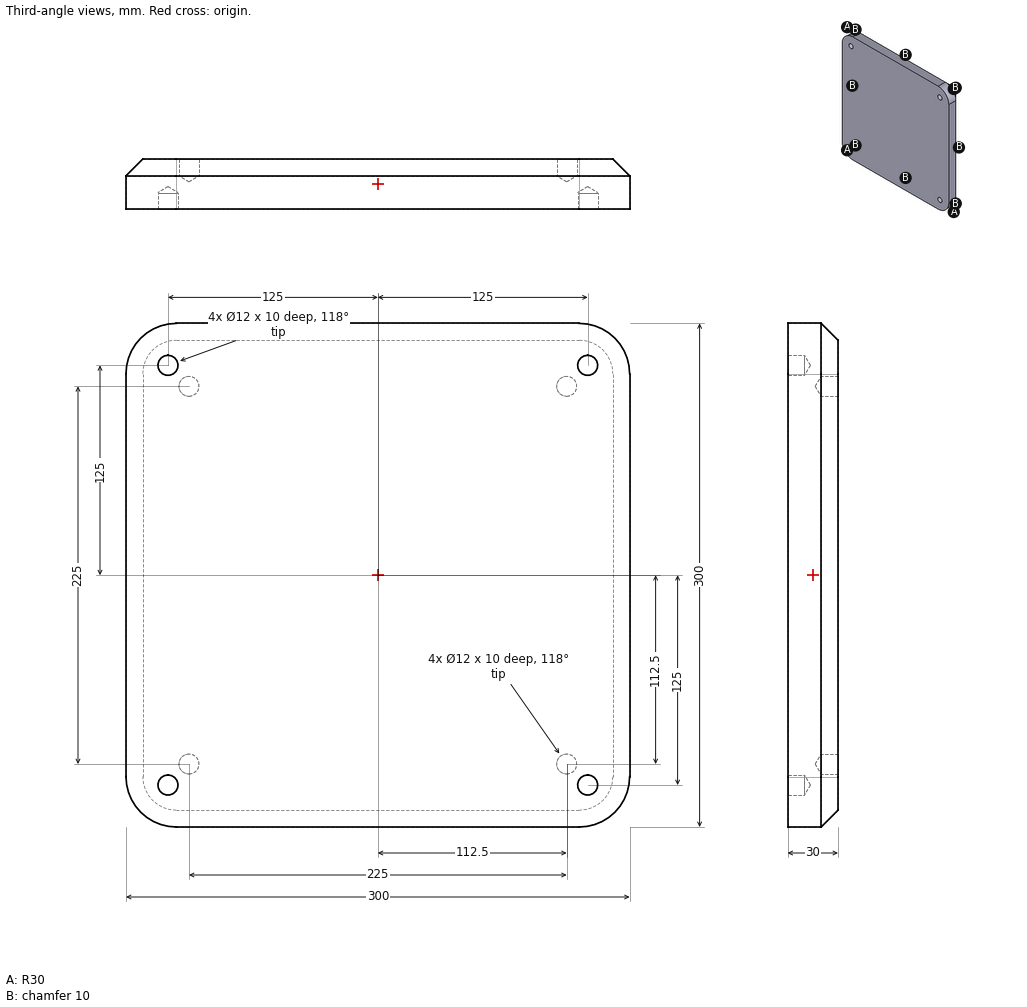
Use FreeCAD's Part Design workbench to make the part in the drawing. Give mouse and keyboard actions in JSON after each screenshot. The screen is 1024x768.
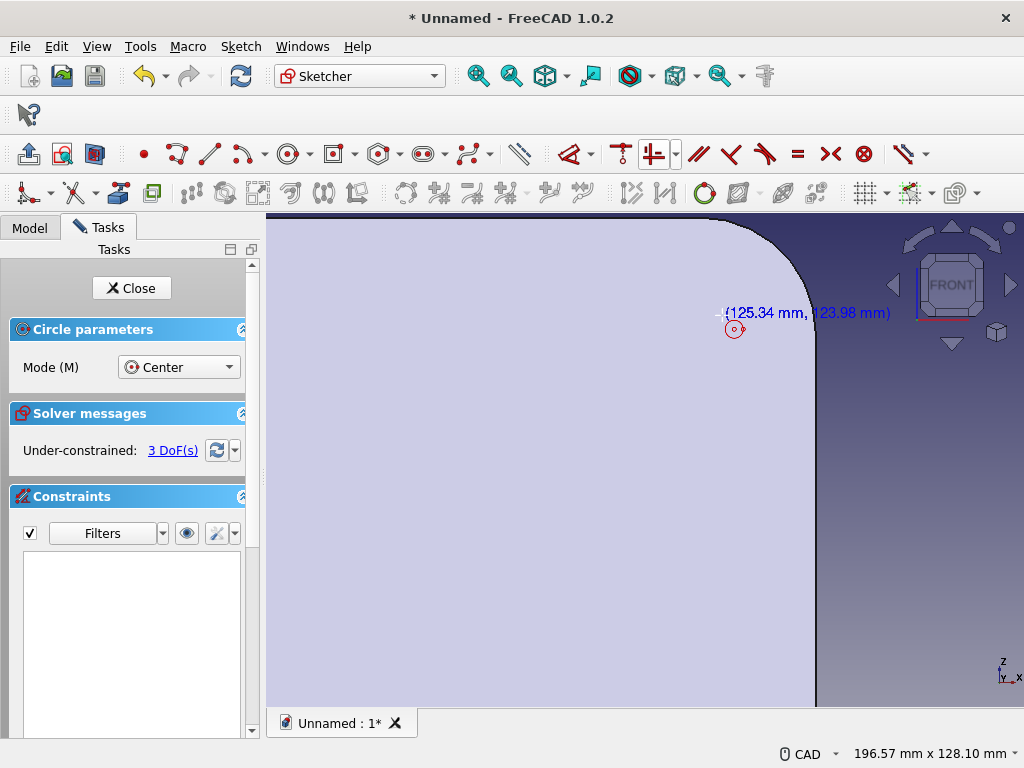
{"action": "left_click", "coordinate": [719, 314]}
{"action": "left_click", "coordinate": [736, 298]}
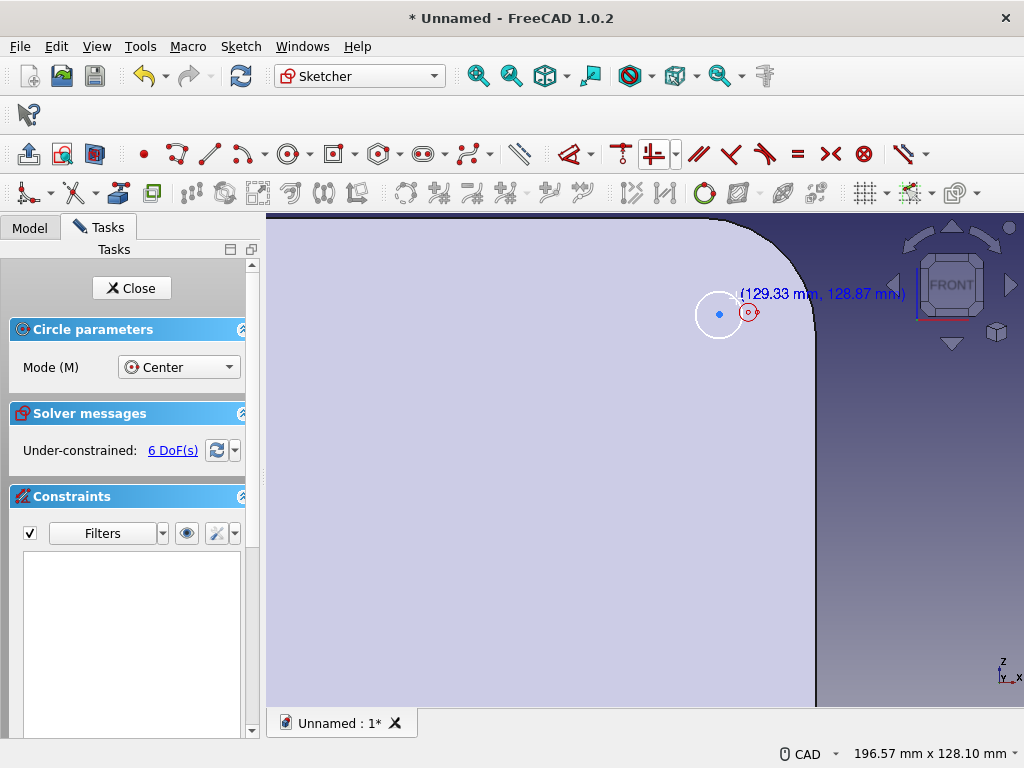
{"action": "scroll", "coordinate": [723, 315], "scroll_direction": "down", "scroll_amount": 6}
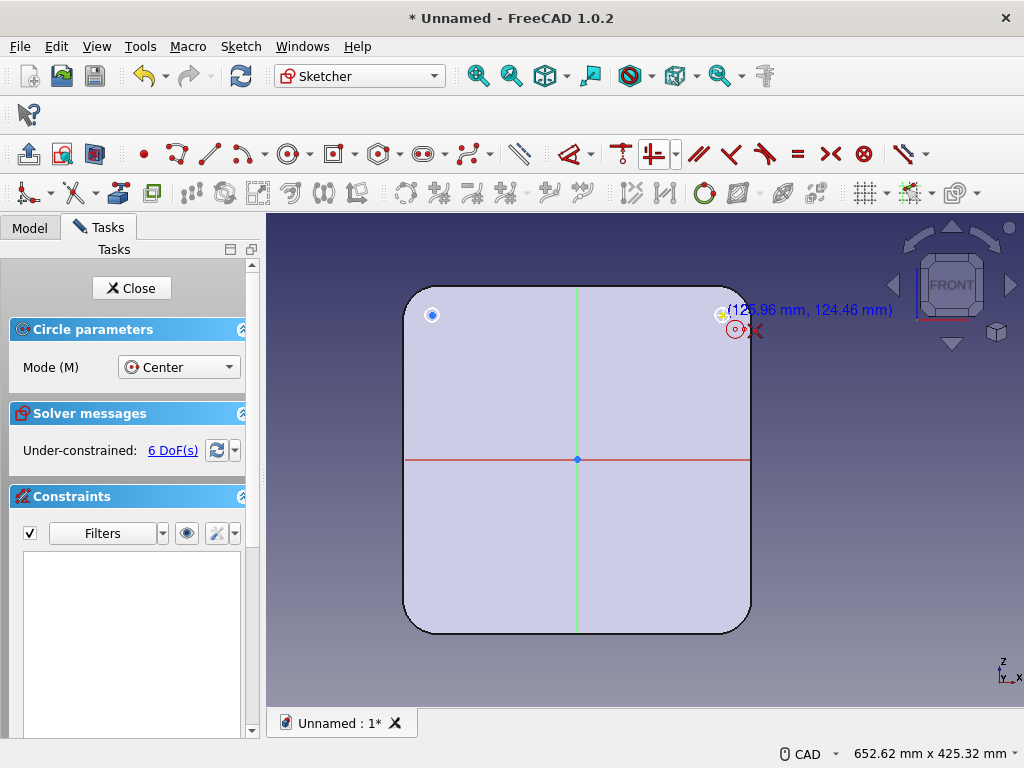
{"action": "scroll", "coordinate": [722, 605], "scroll_direction": "up", "scroll_amount": 6}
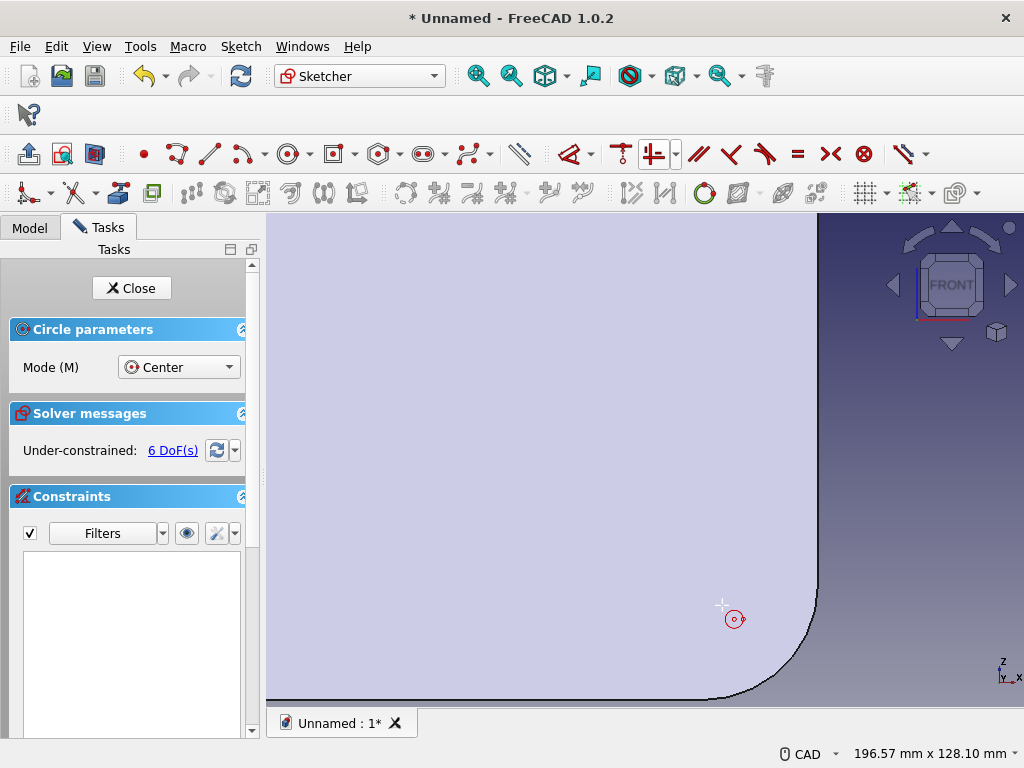
{"action": "left_click", "coordinate": [722, 604]}
{"action": "left_click", "coordinate": [738, 587]}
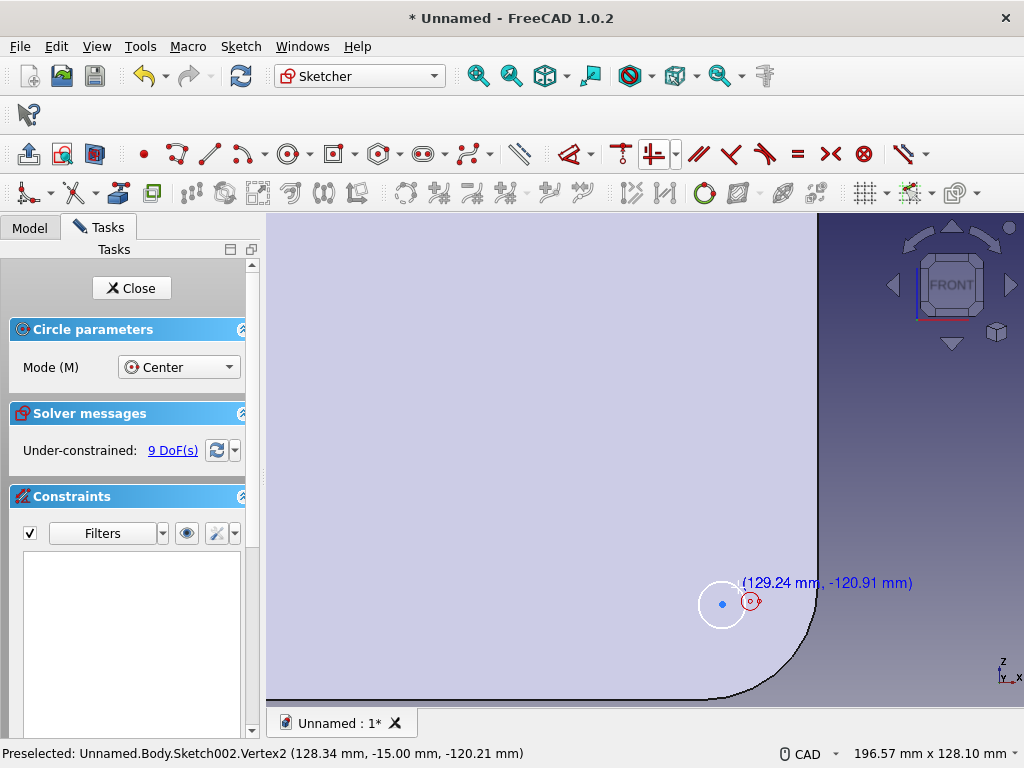
{"action": "scroll", "coordinate": [722, 606], "scroll_direction": "down", "scroll_amount": 6}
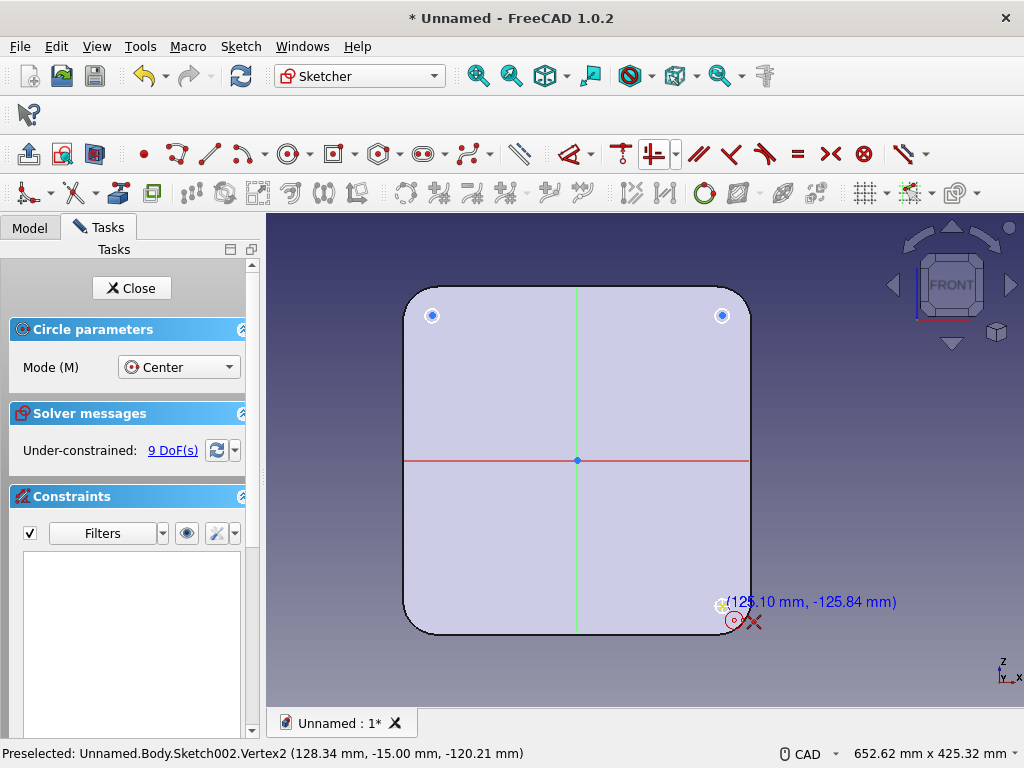
{"action": "scroll", "coordinate": [432, 606], "scroll_direction": "up", "scroll_amount": 6}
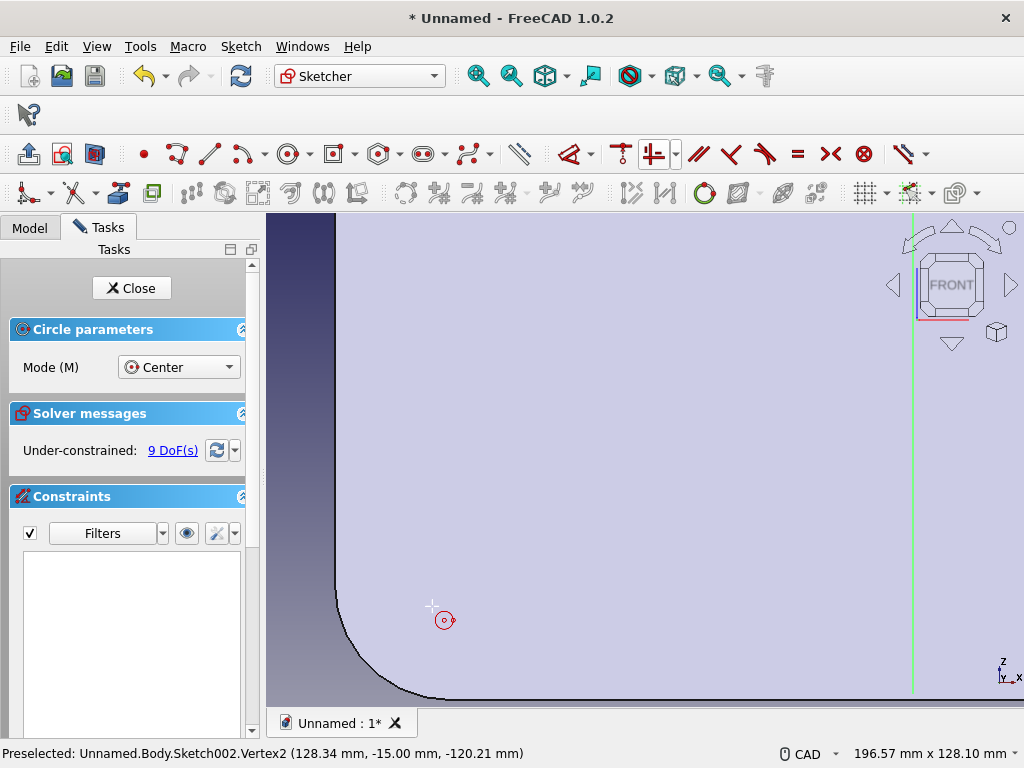
{"action": "left_click", "coordinate": [431, 604]}
{"action": "left_click", "coordinate": [448, 587]}
{"action": "key", "text": "Escape"}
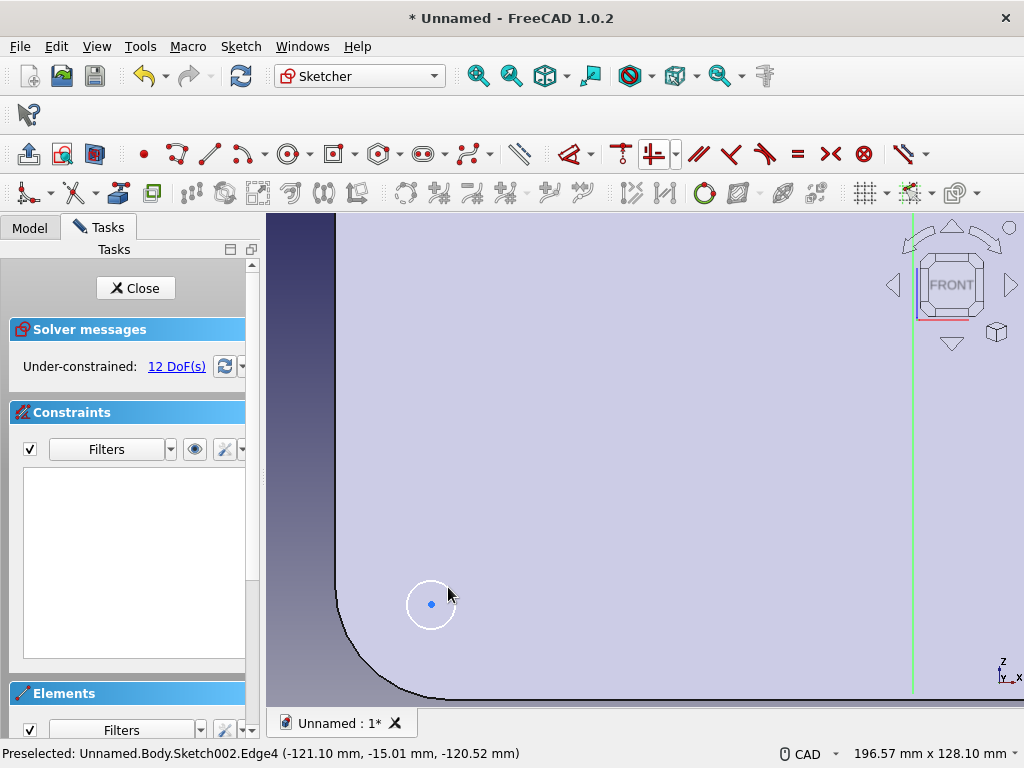
{"action": "scroll", "coordinate": [431, 606], "scroll_direction": "down", "scroll_amount": 6}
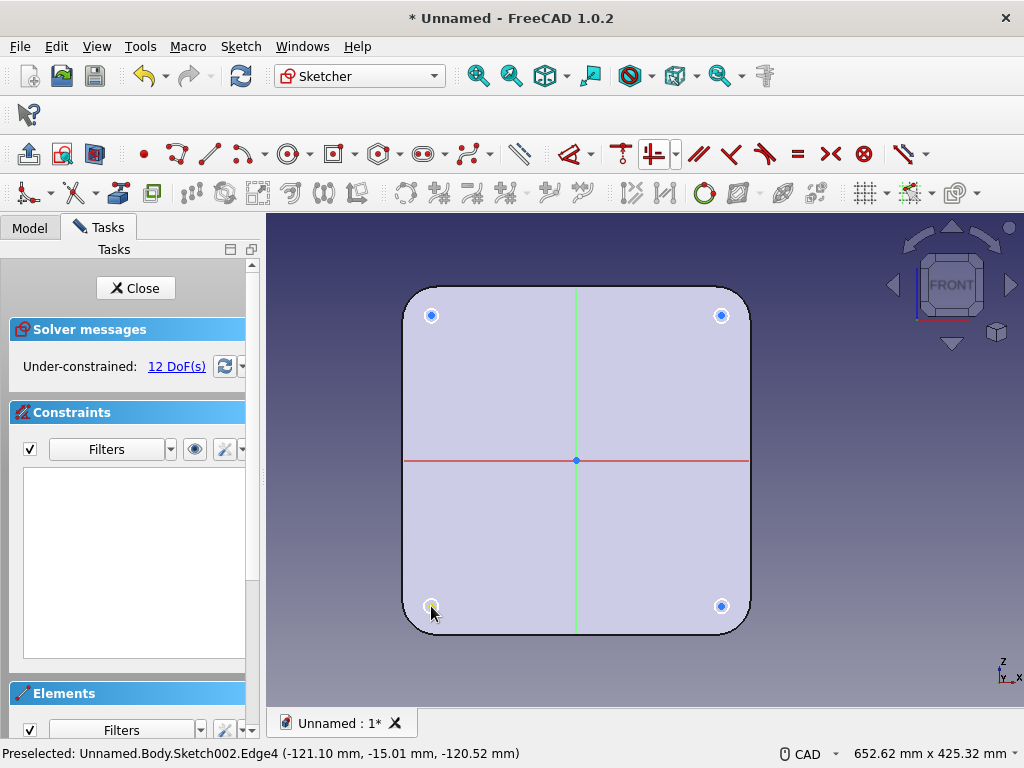
{"action": "scroll", "coordinate": [436, 311], "scroll_direction": "up", "scroll_amount": 4}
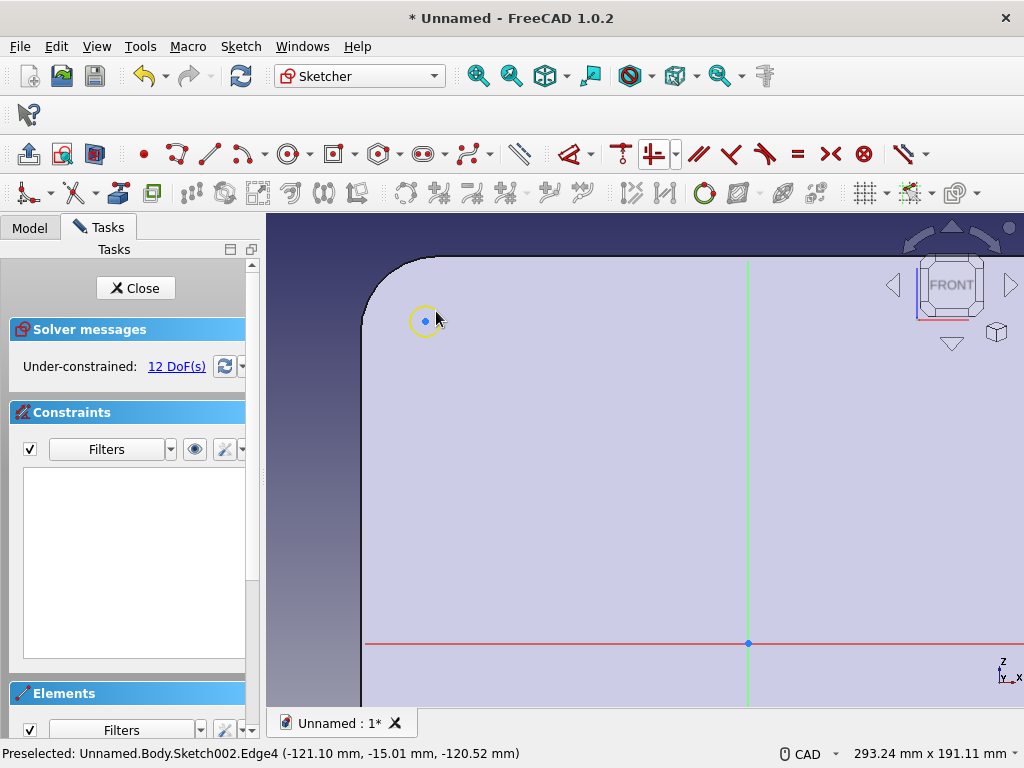
{"action": "left_click", "coordinate": [436, 311]}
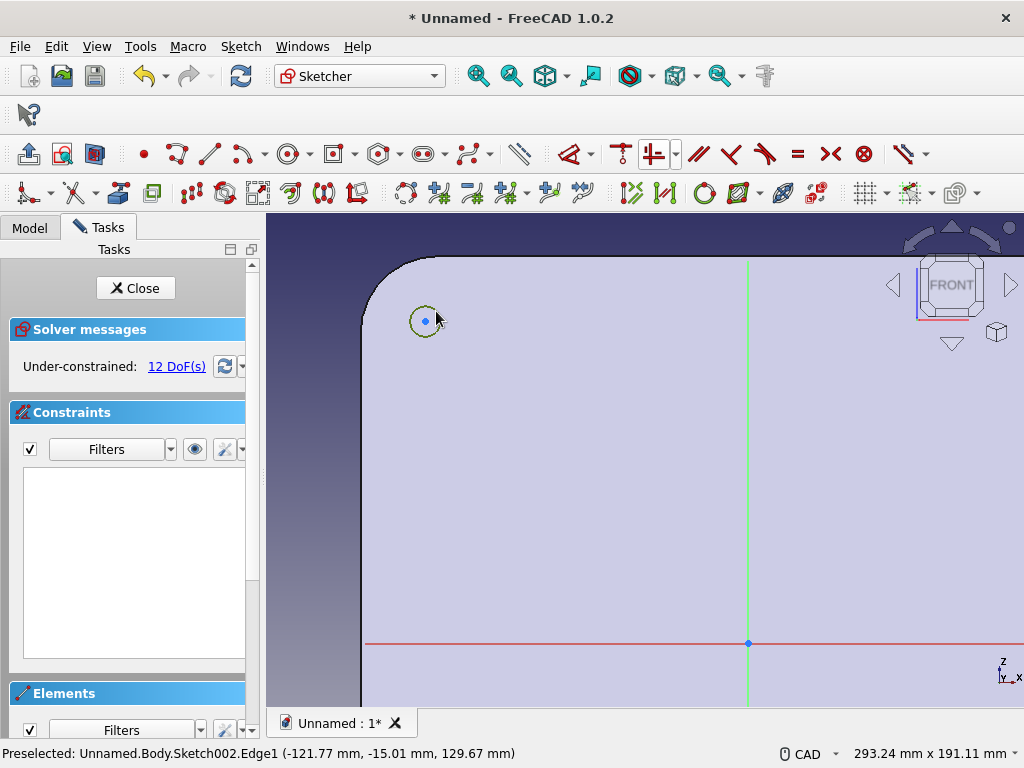
{"action": "scroll", "coordinate": [436, 310], "scroll_direction": "down", "scroll_amount": 4}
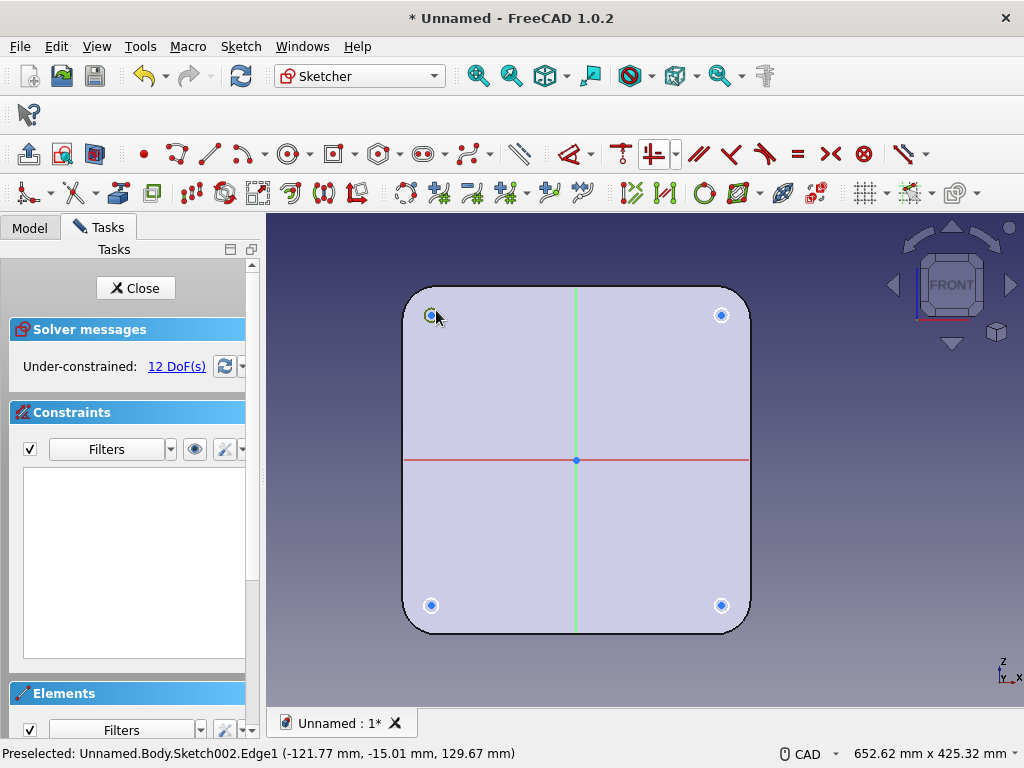
{"action": "scroll", "coordinate": [726, 310], "scroll_direction": "up", "scroll_amount": 4}